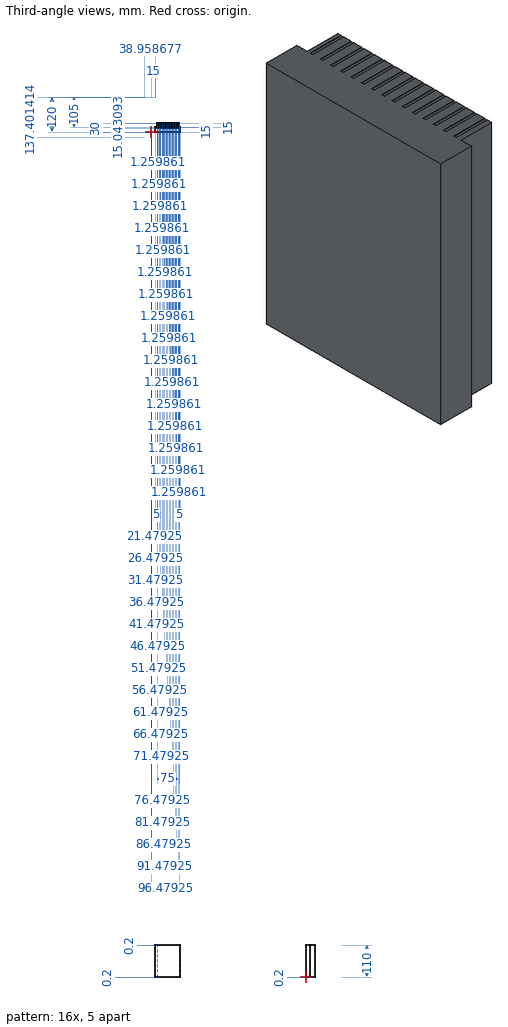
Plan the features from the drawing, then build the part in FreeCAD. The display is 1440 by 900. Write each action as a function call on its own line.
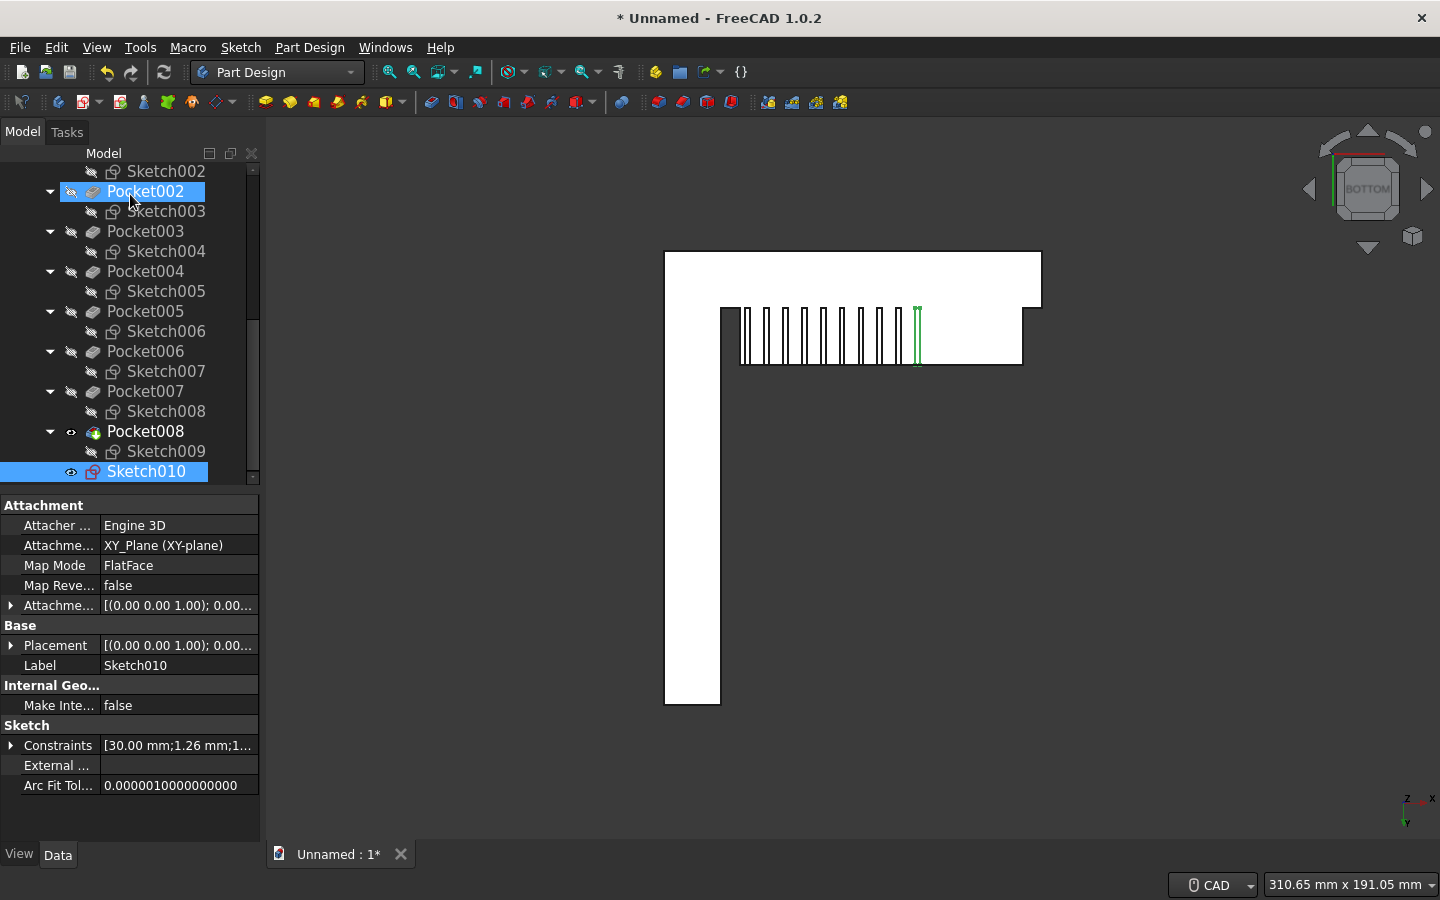
click(432, 102)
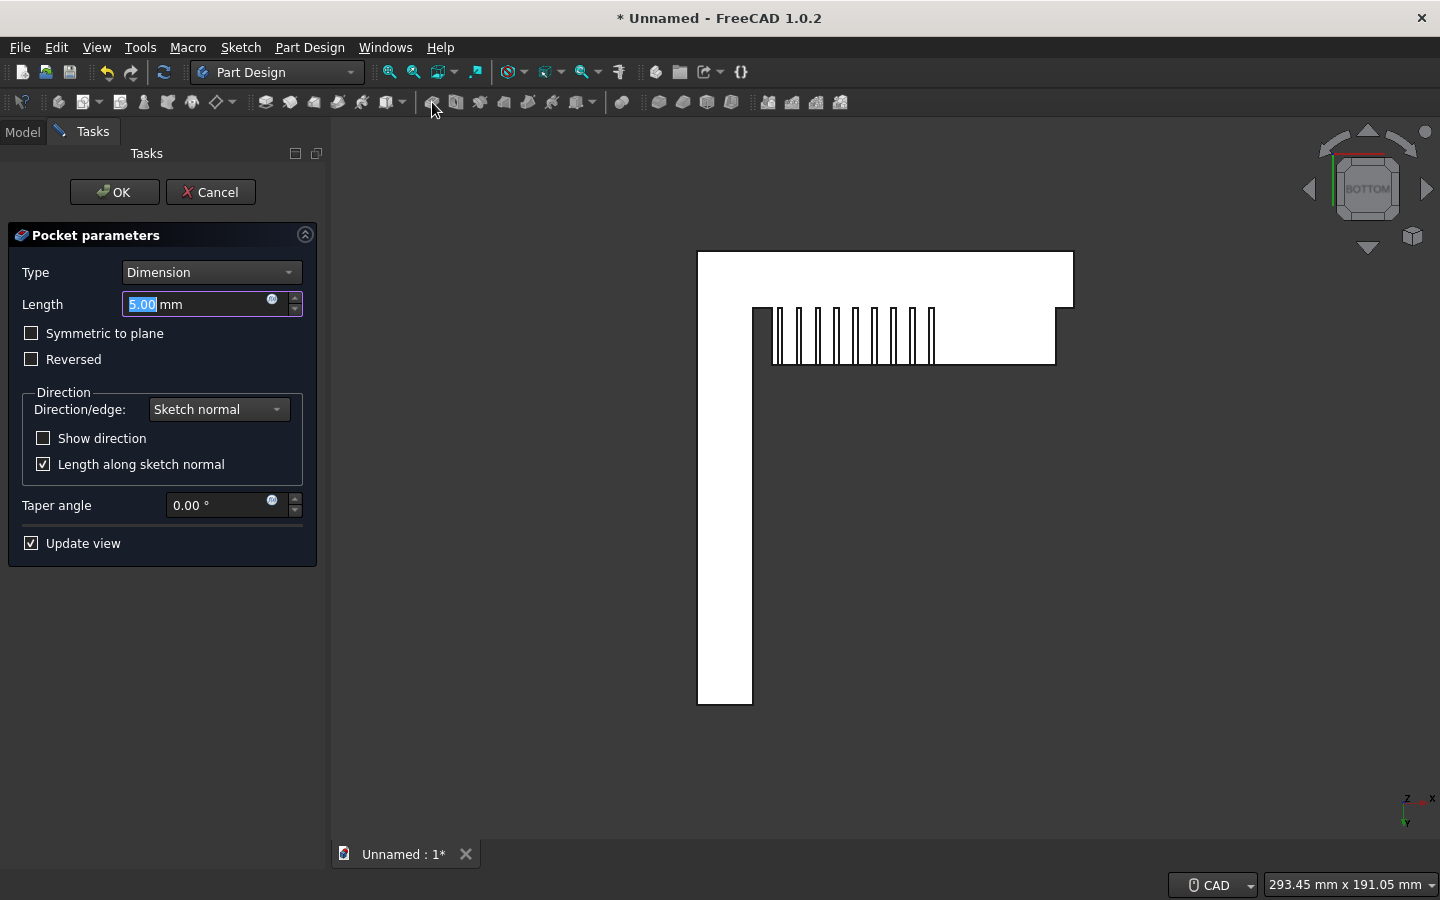
text(0.2)
key(Tab)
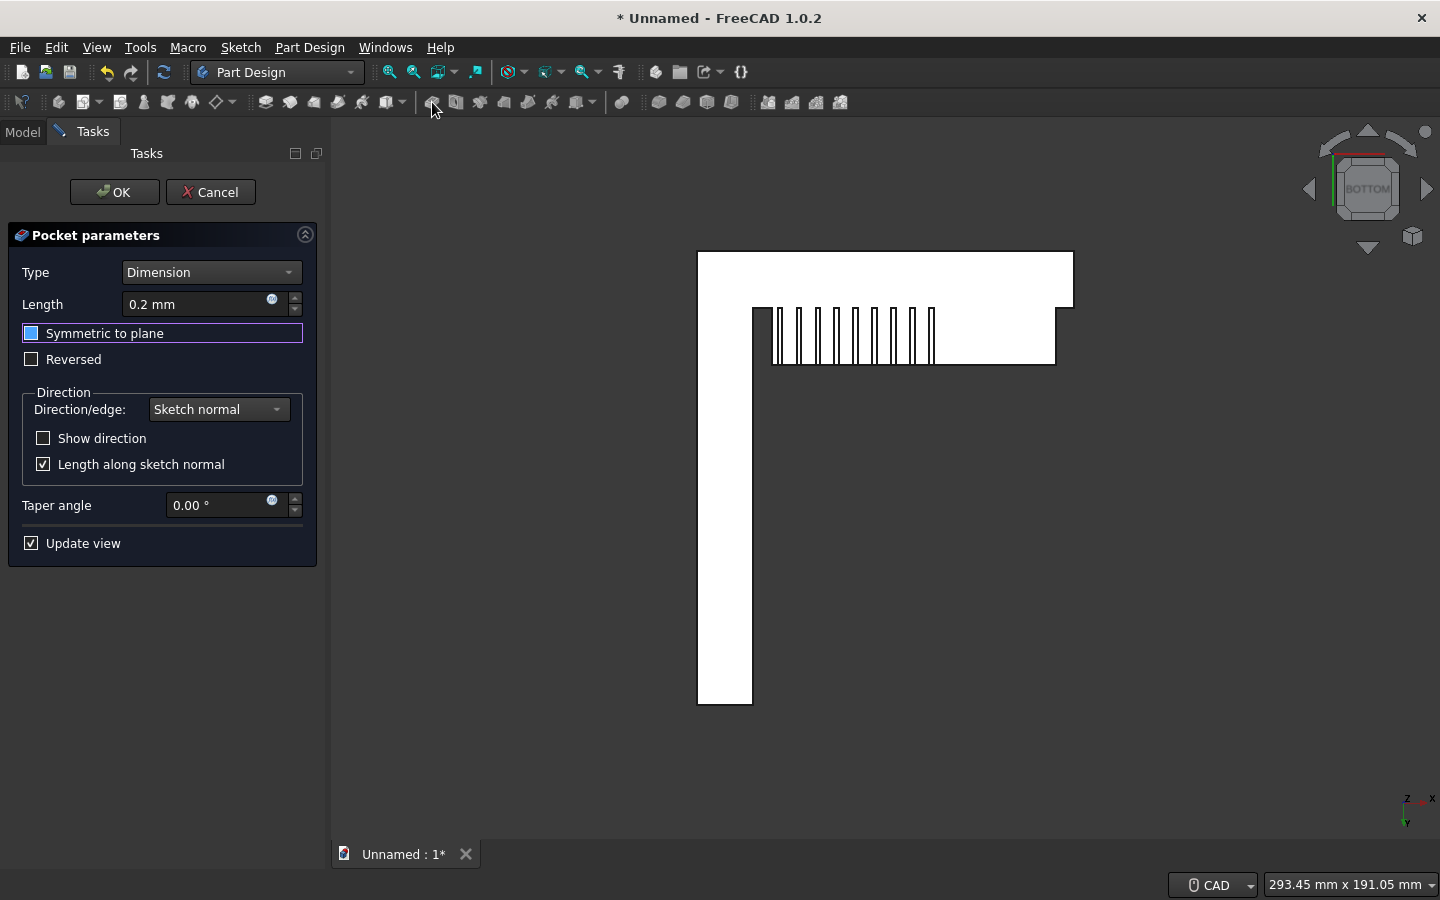
click(30, 359)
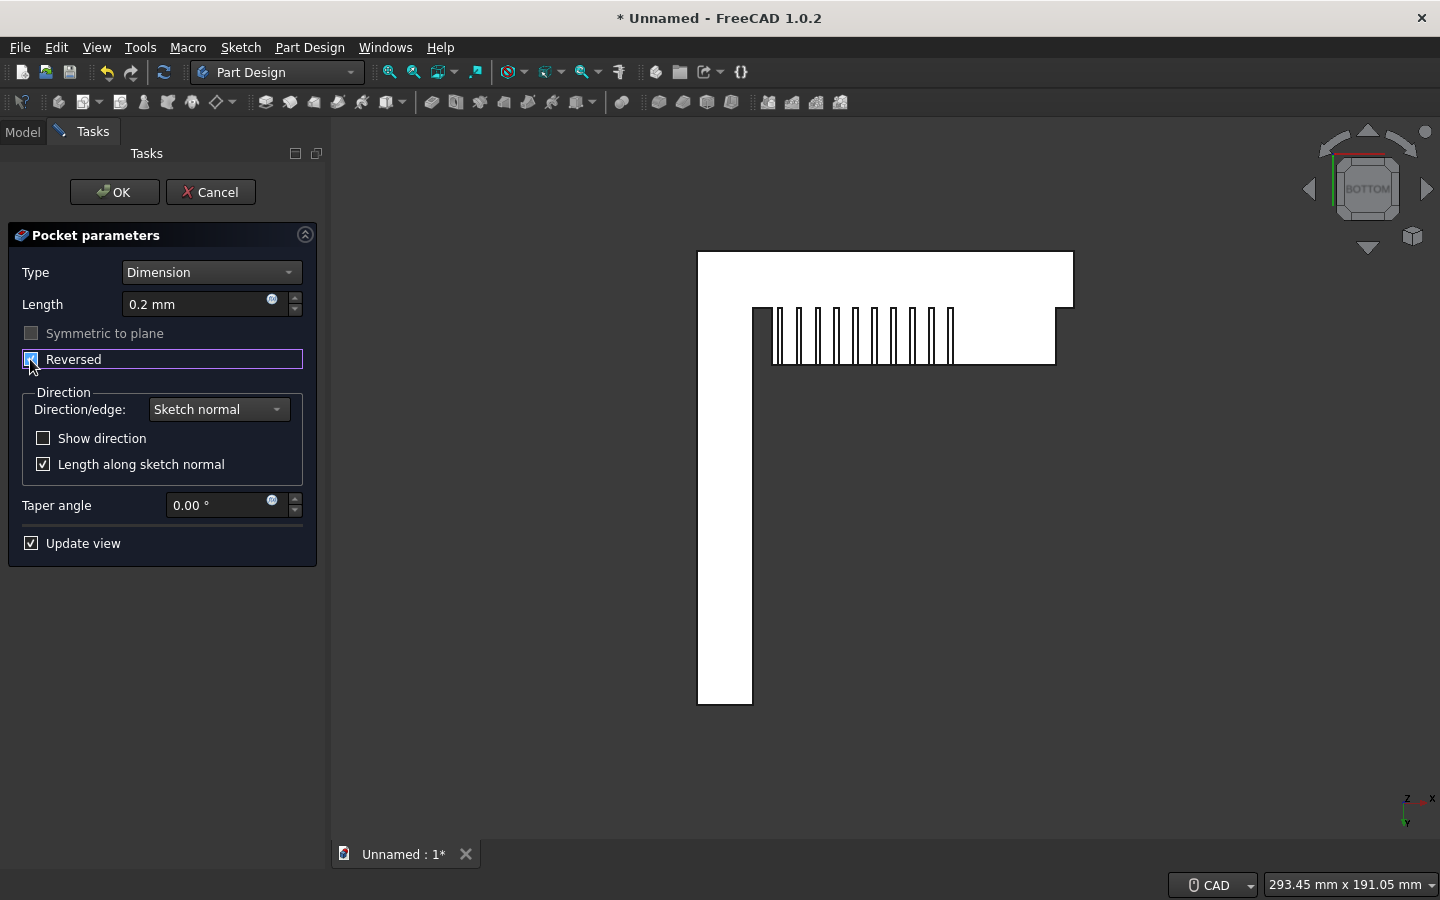
click(115, 192)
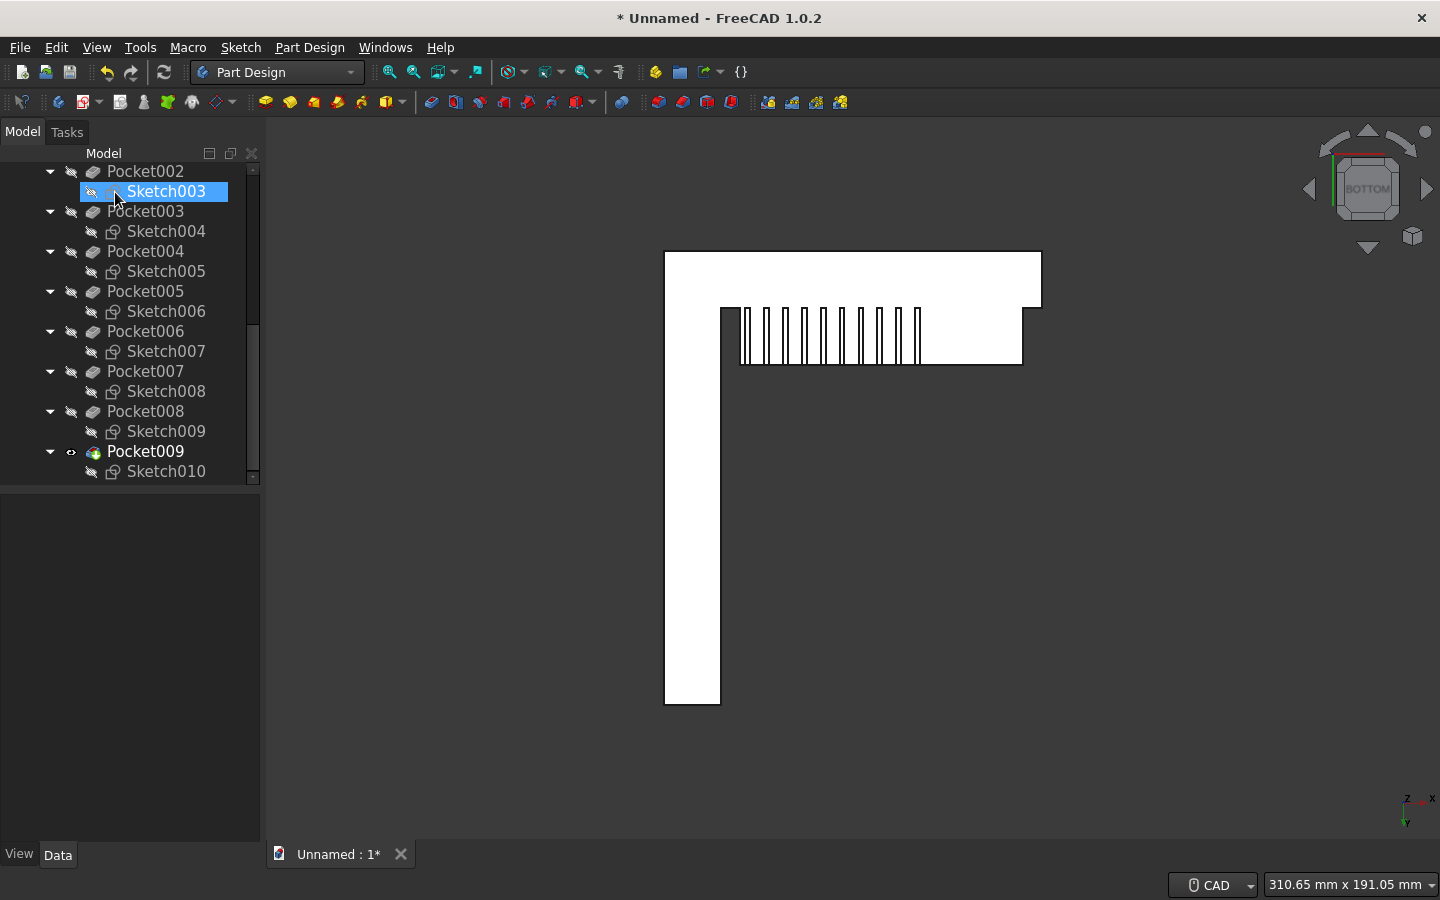
click(84, 102)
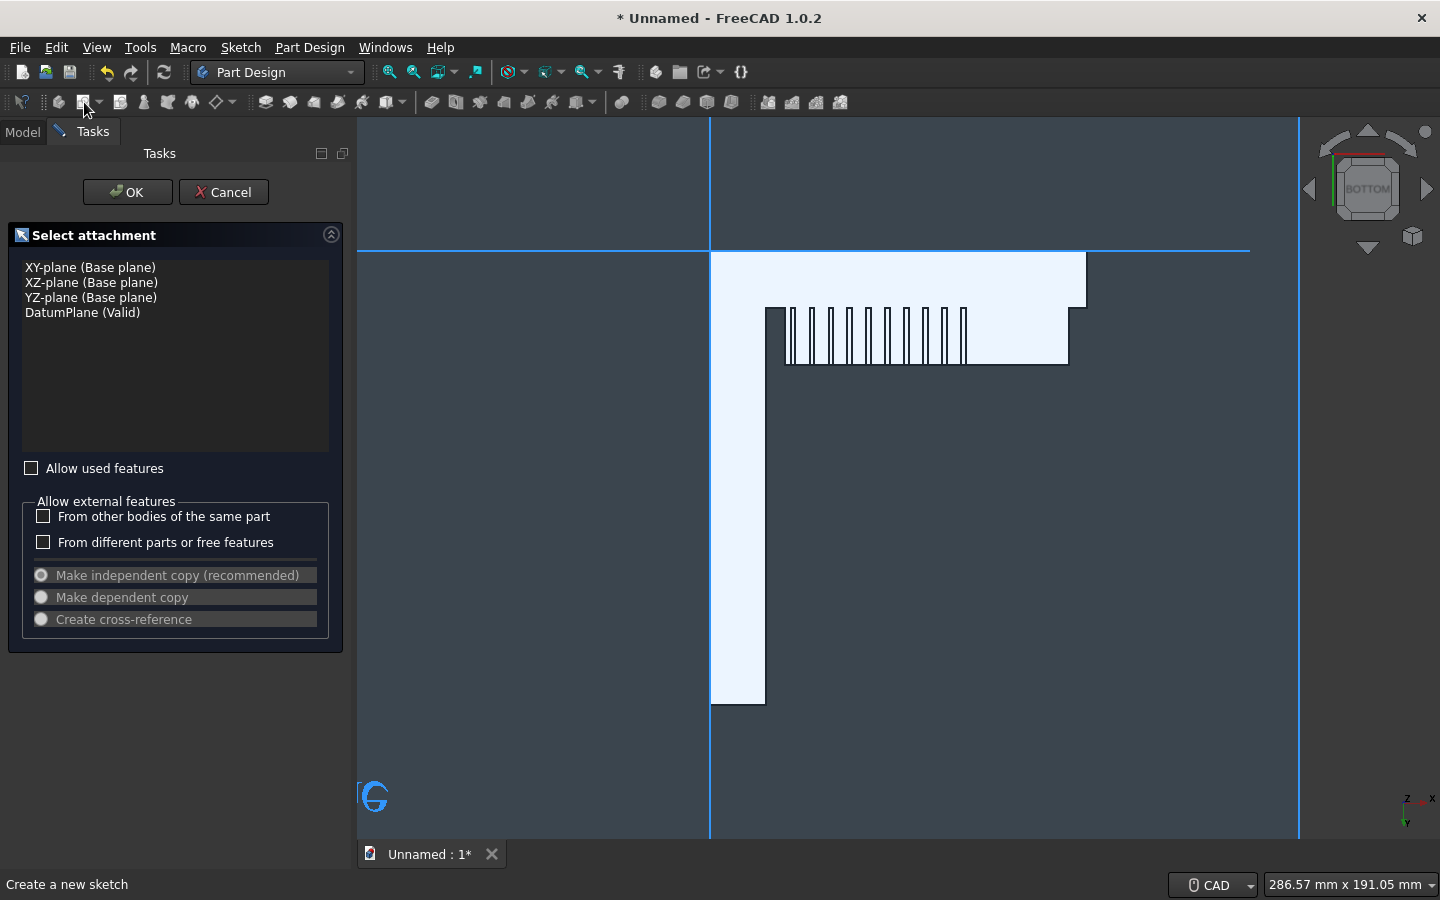
click(82, 268)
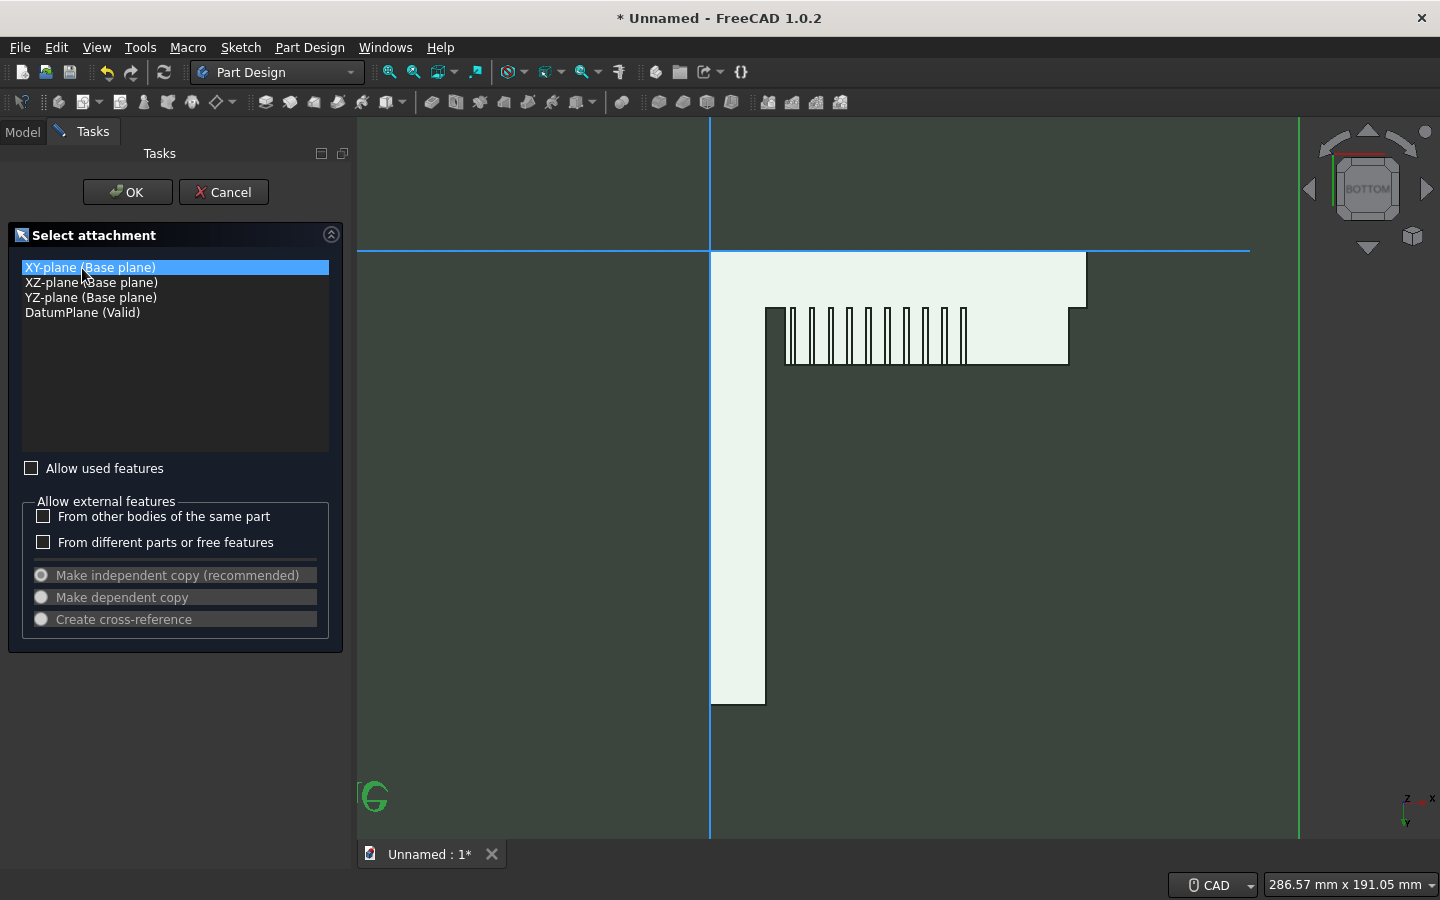
click(128, 192)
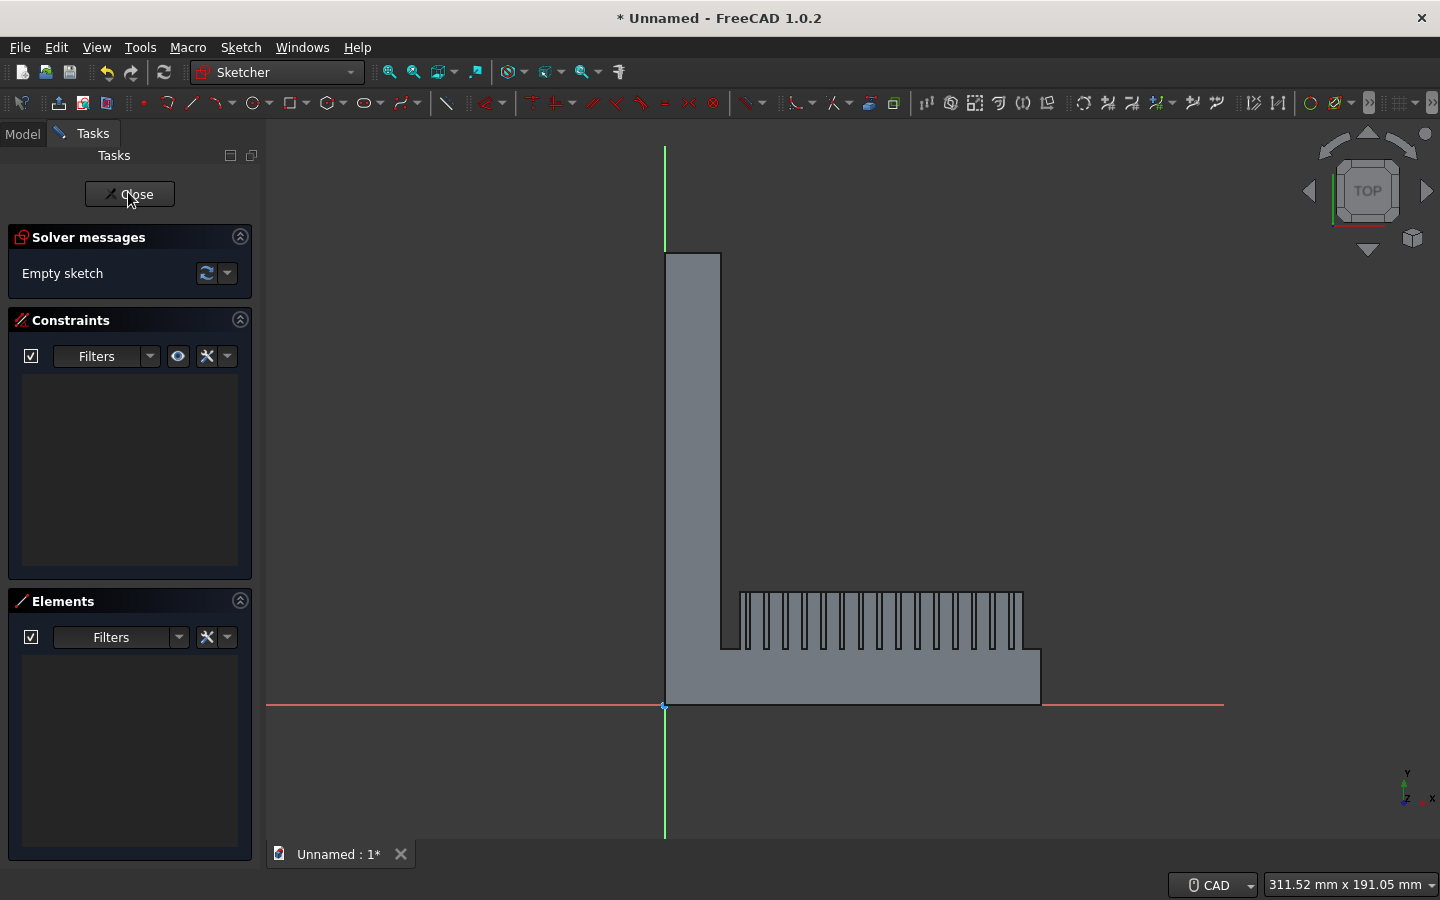
click(108, 104)